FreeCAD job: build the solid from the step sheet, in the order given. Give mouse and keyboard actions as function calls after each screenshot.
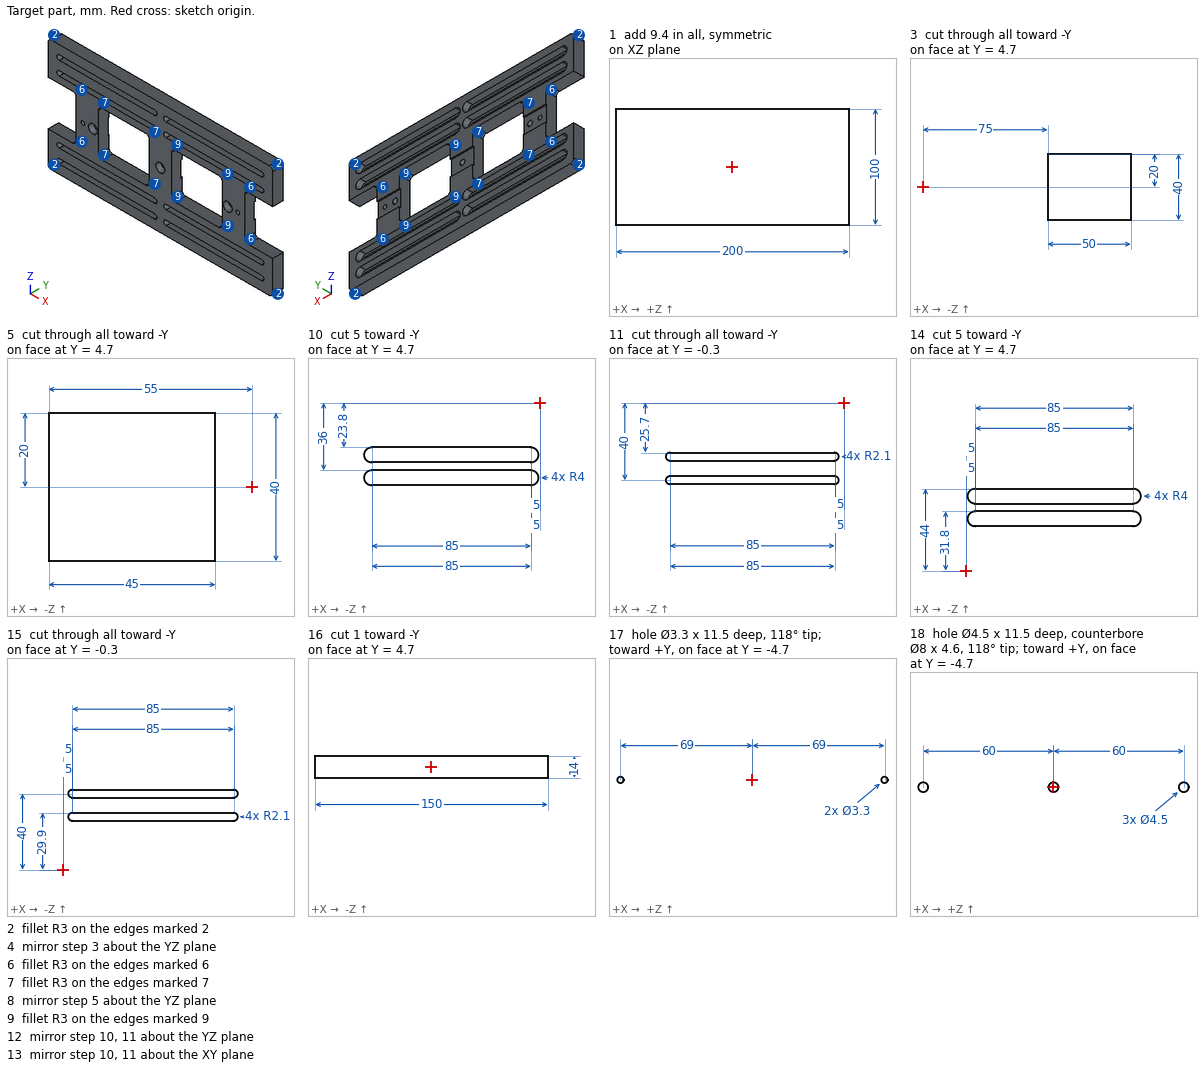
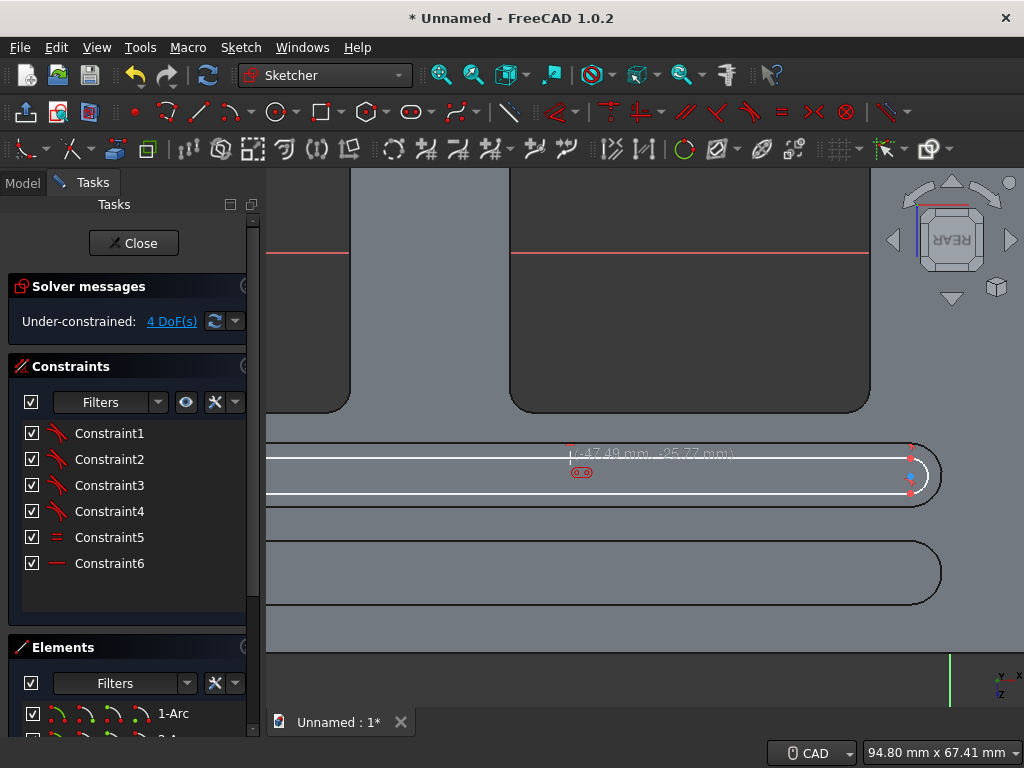
scroll(570, 457, down, 3)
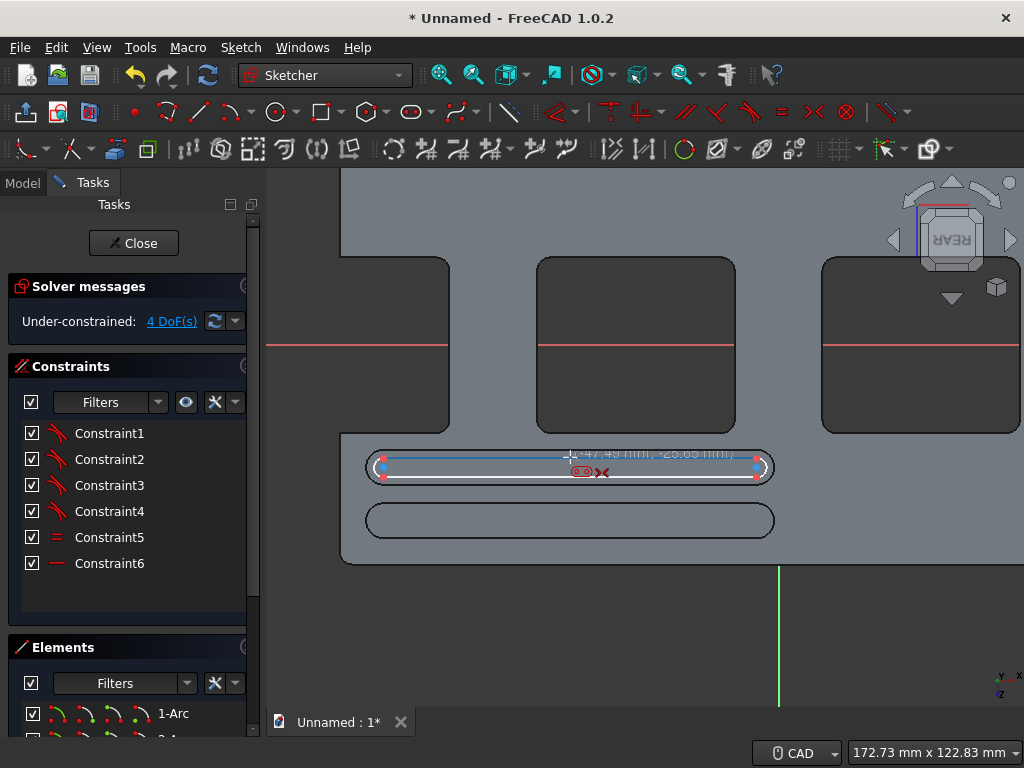
scroll(384, 521, up, 5)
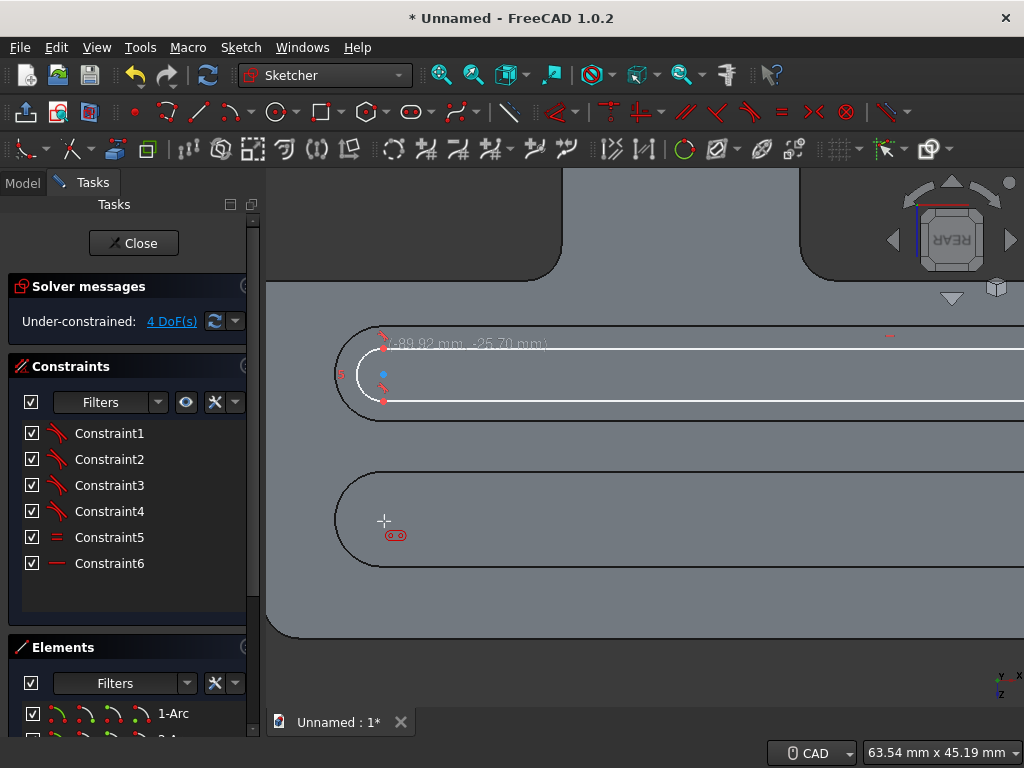
click(383, 519)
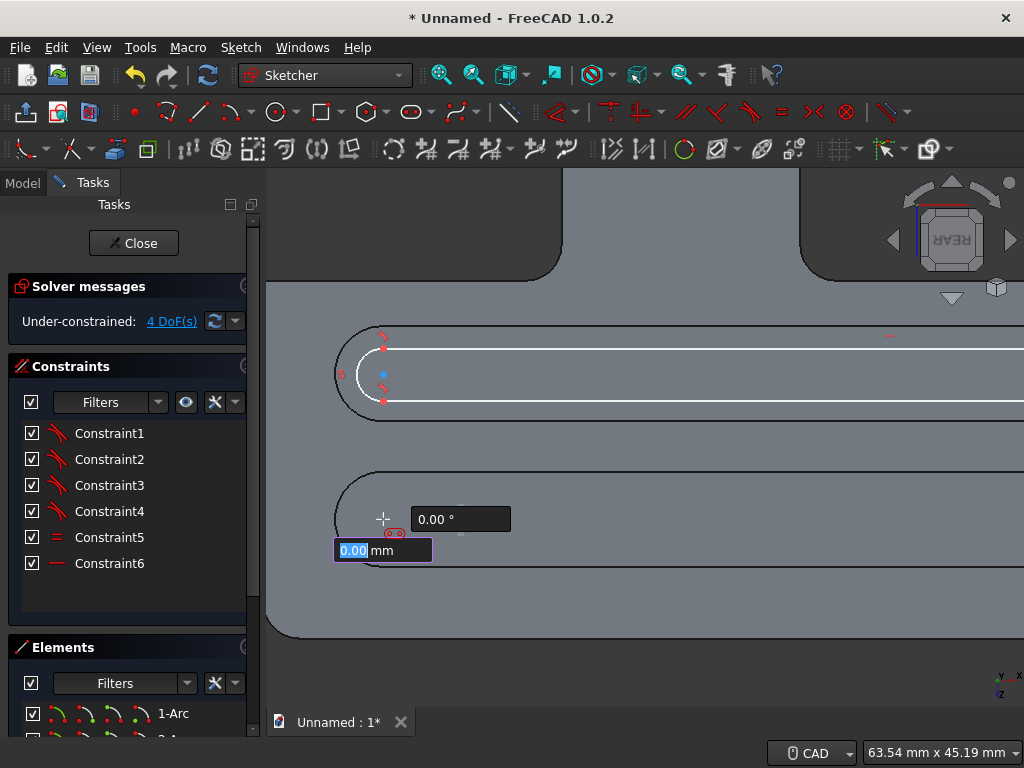
scroll(384, 521, down, 5)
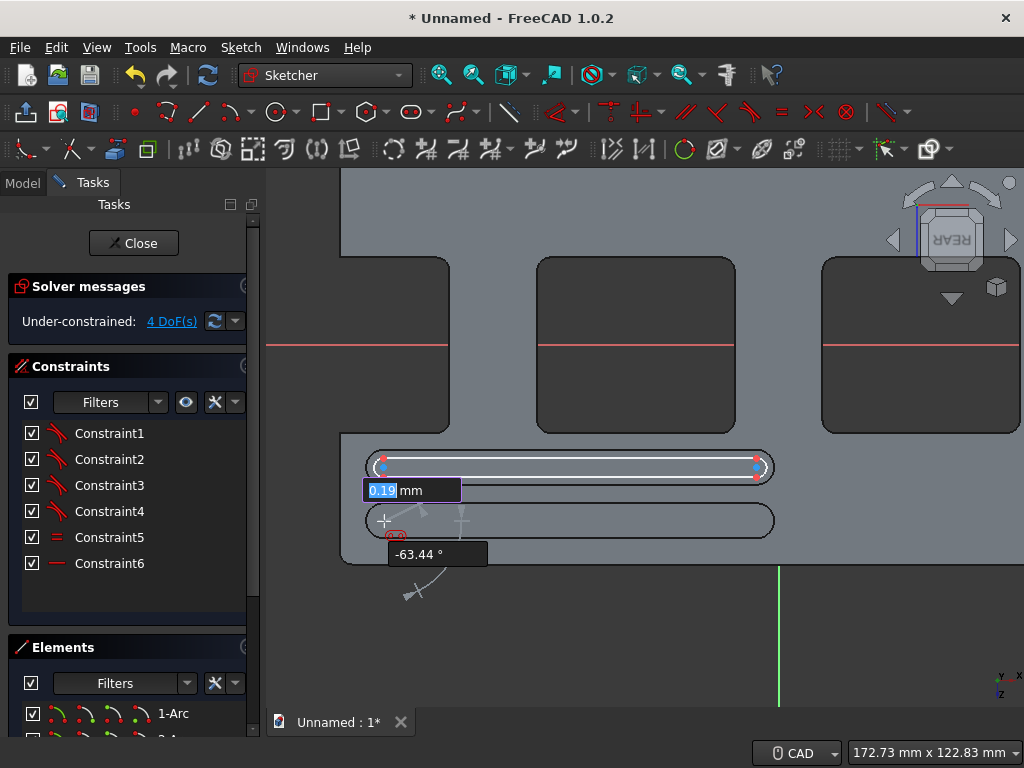
click(757, 521)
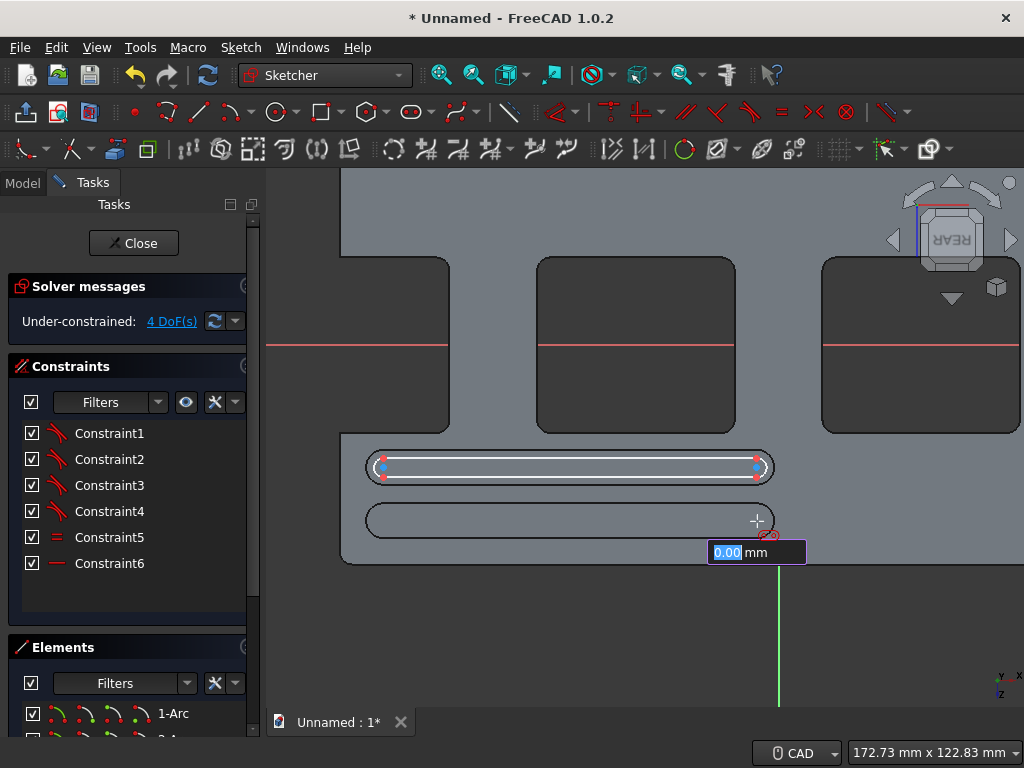
scroll(570, 512, up, 3)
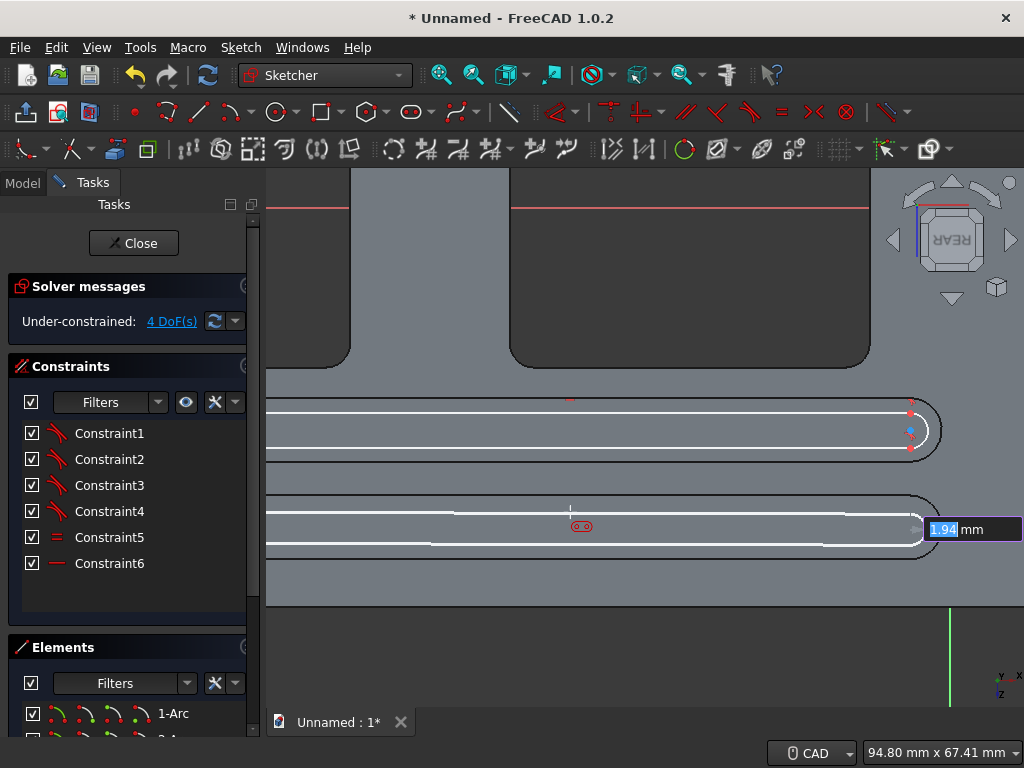
click(570, 511)
key(Escape)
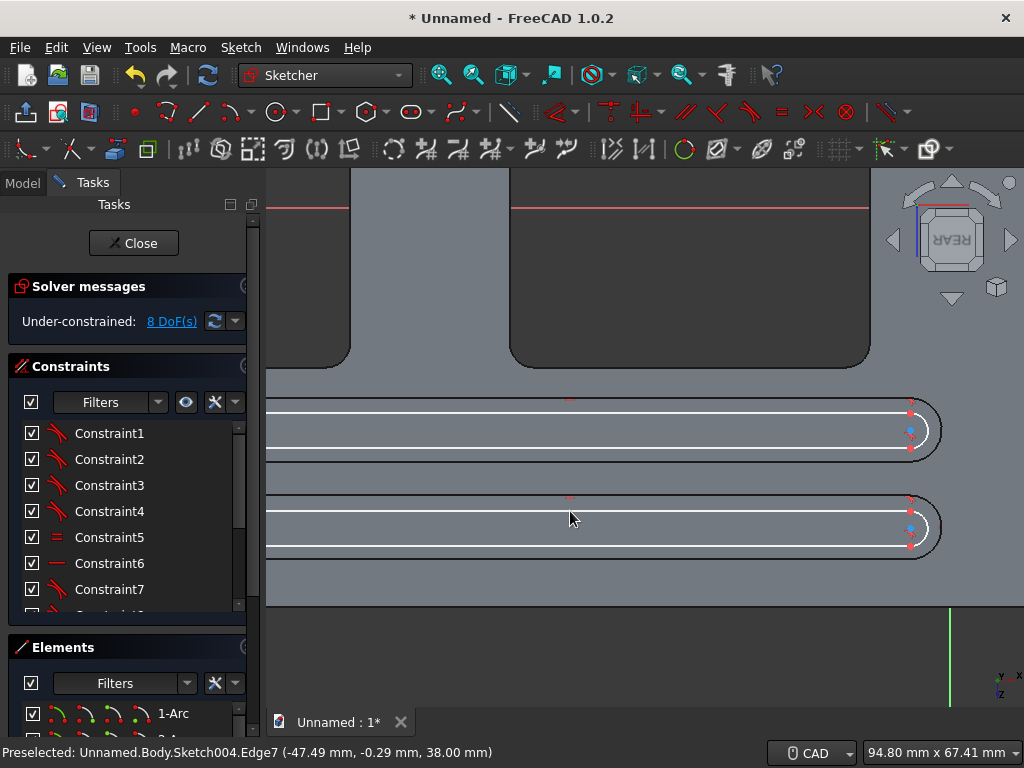
scroll(570, 512, down, 3)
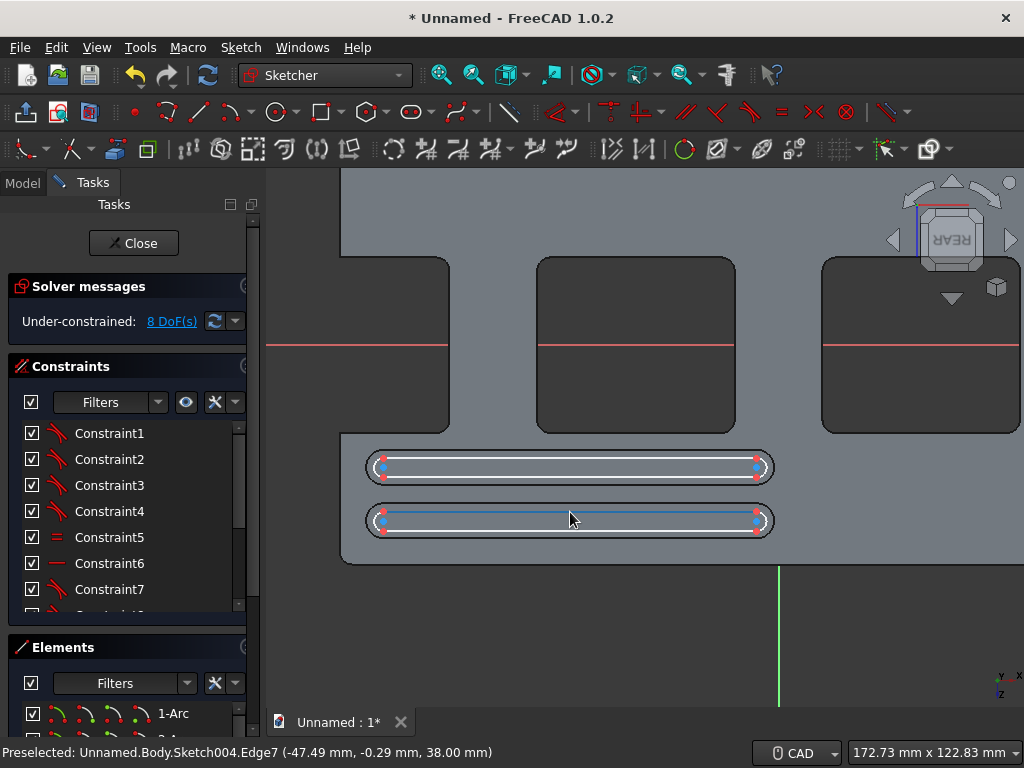
scroll(376, 462, up, 3)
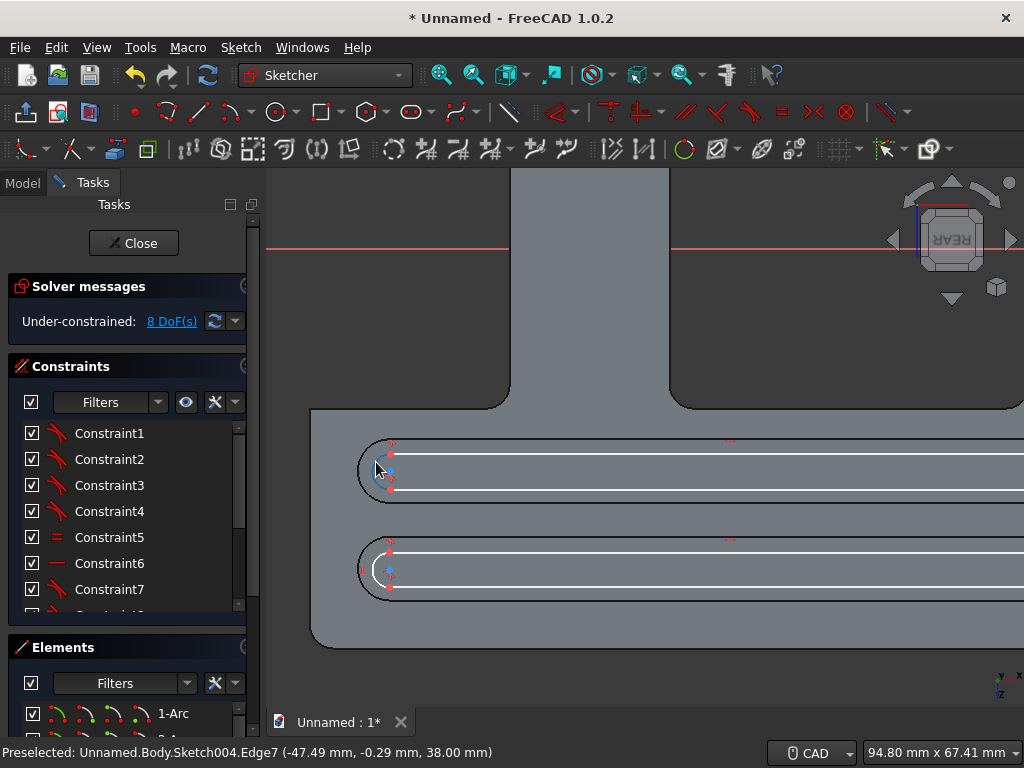
click(376, 462)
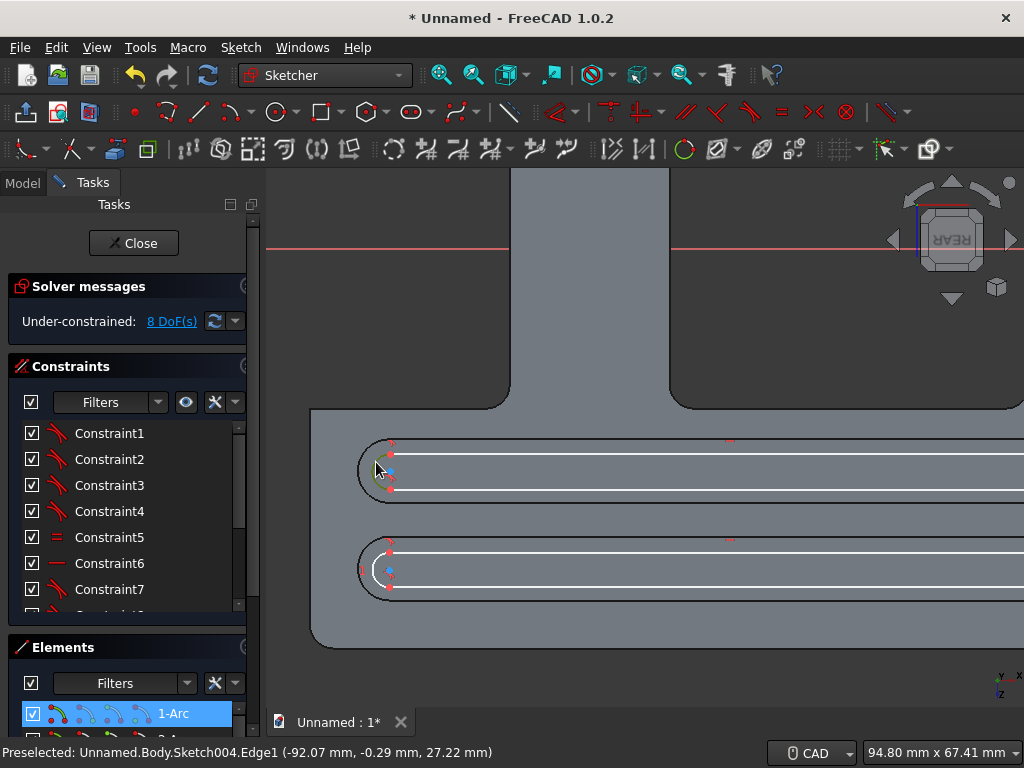
click(376, 560)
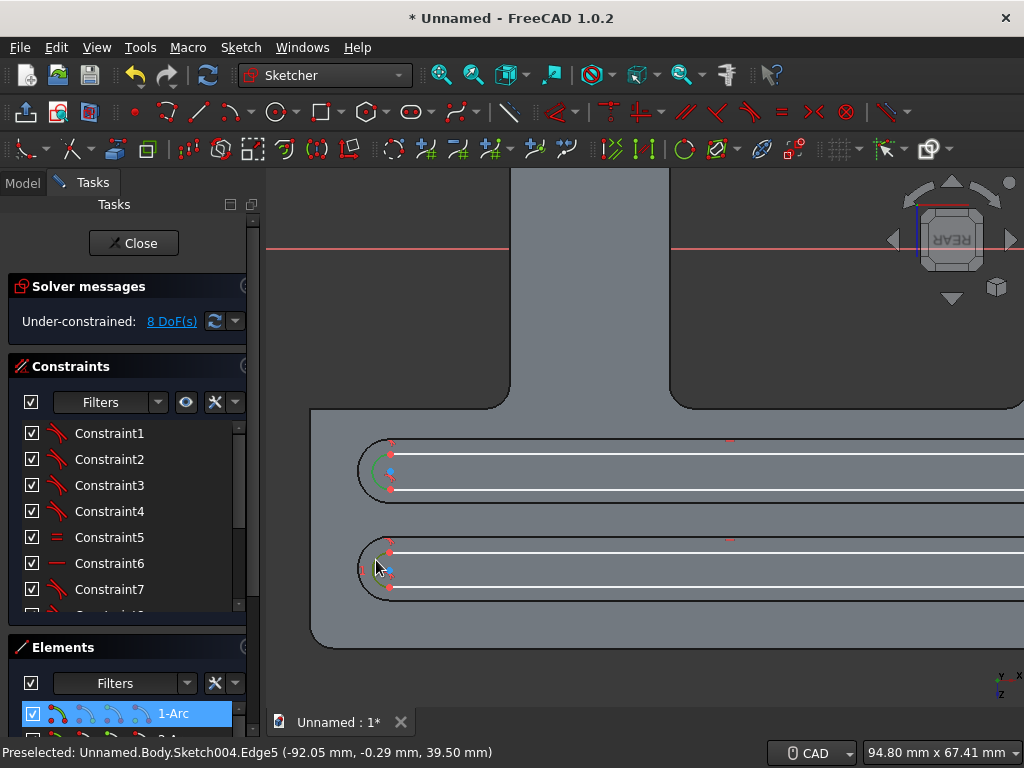
click(782, 112)